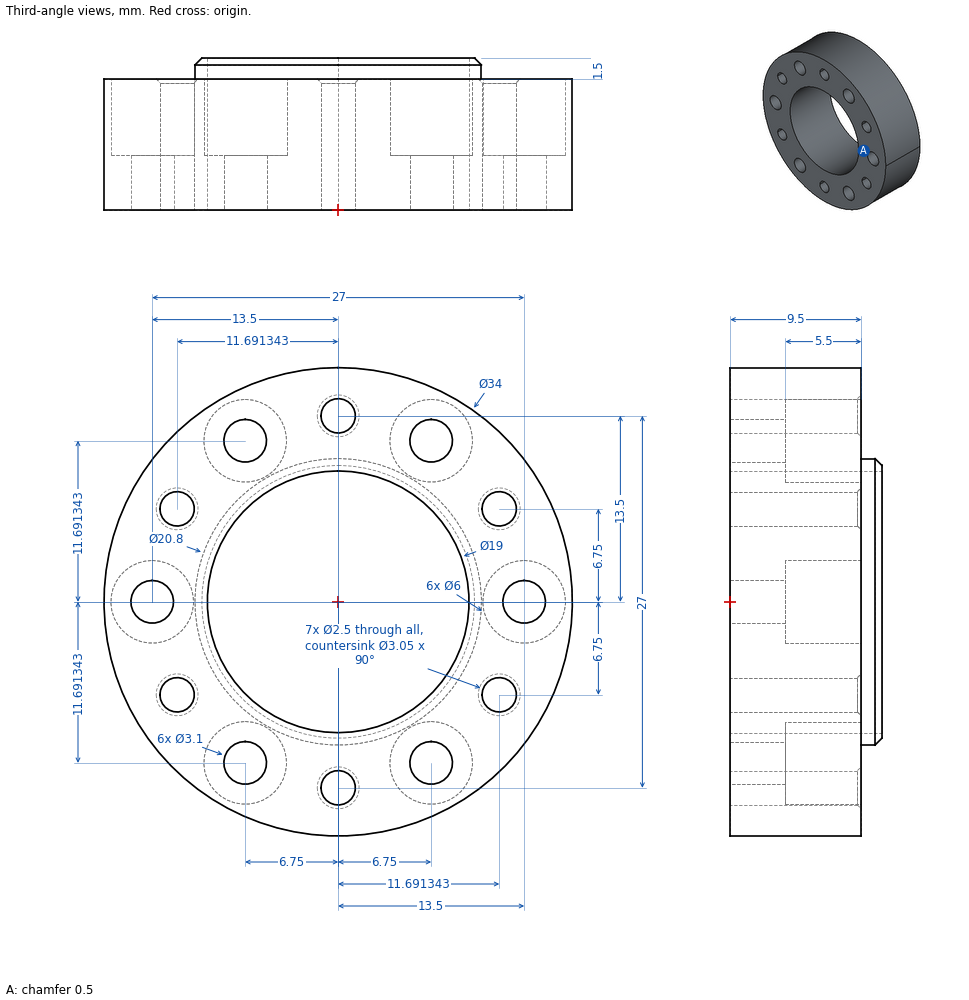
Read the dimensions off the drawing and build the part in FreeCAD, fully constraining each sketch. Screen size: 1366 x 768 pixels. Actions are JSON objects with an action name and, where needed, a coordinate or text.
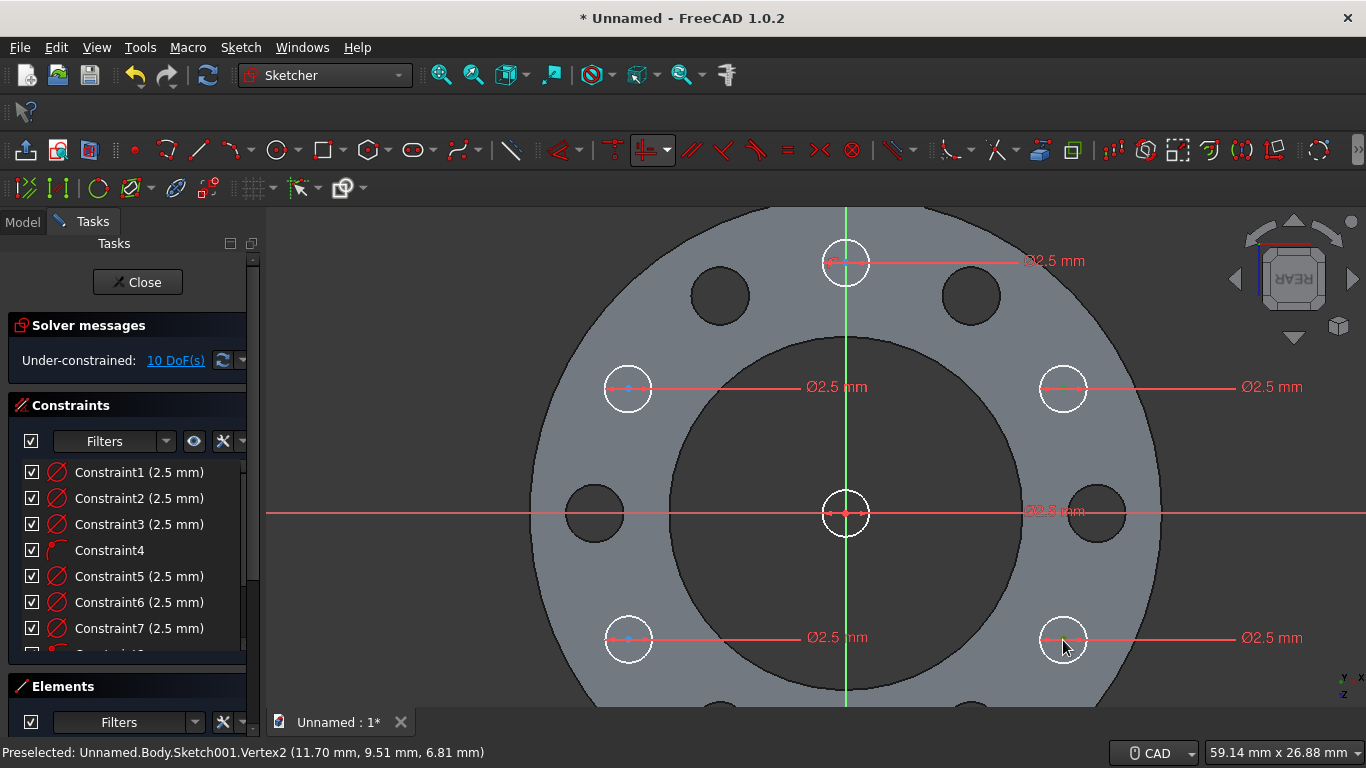
{"action": "left_click", "coordinate": [670, 150]}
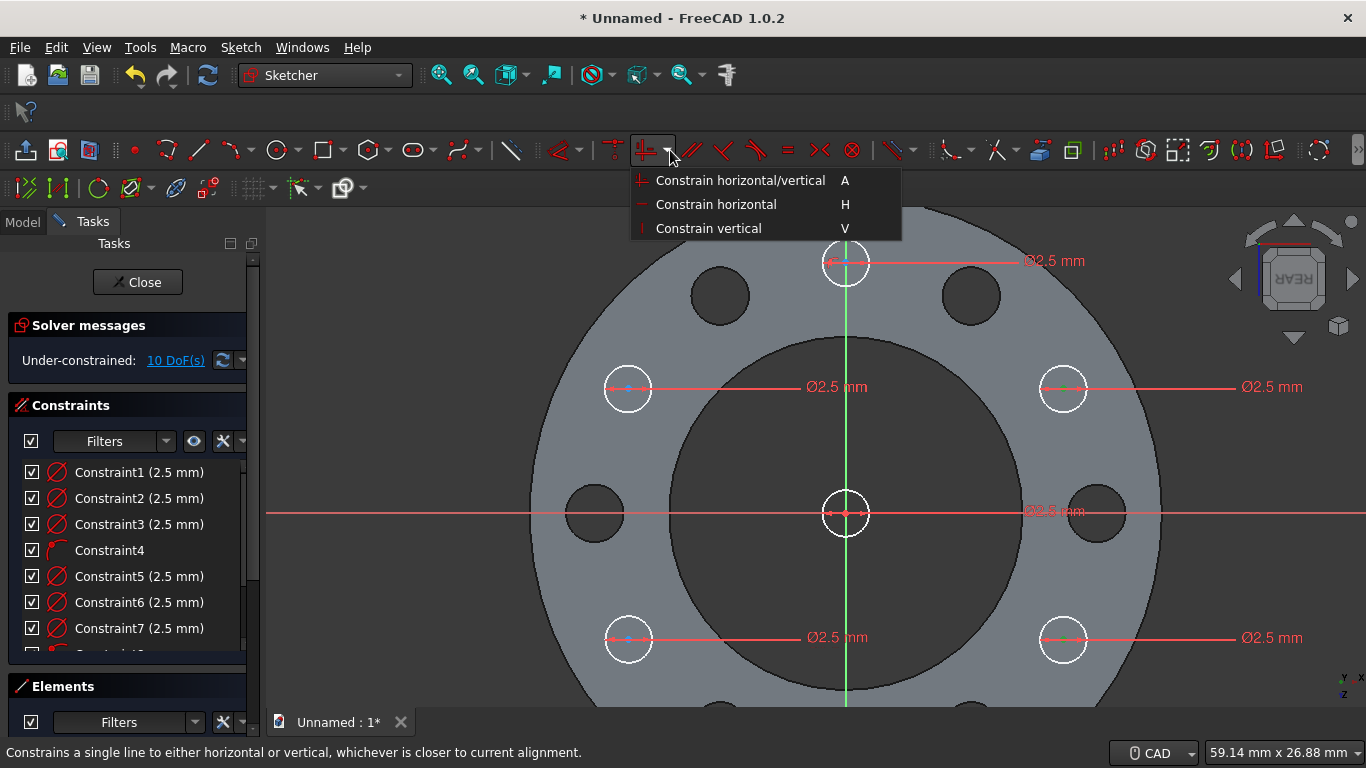
{"action": "left_click", "coordinate": [766, 228]}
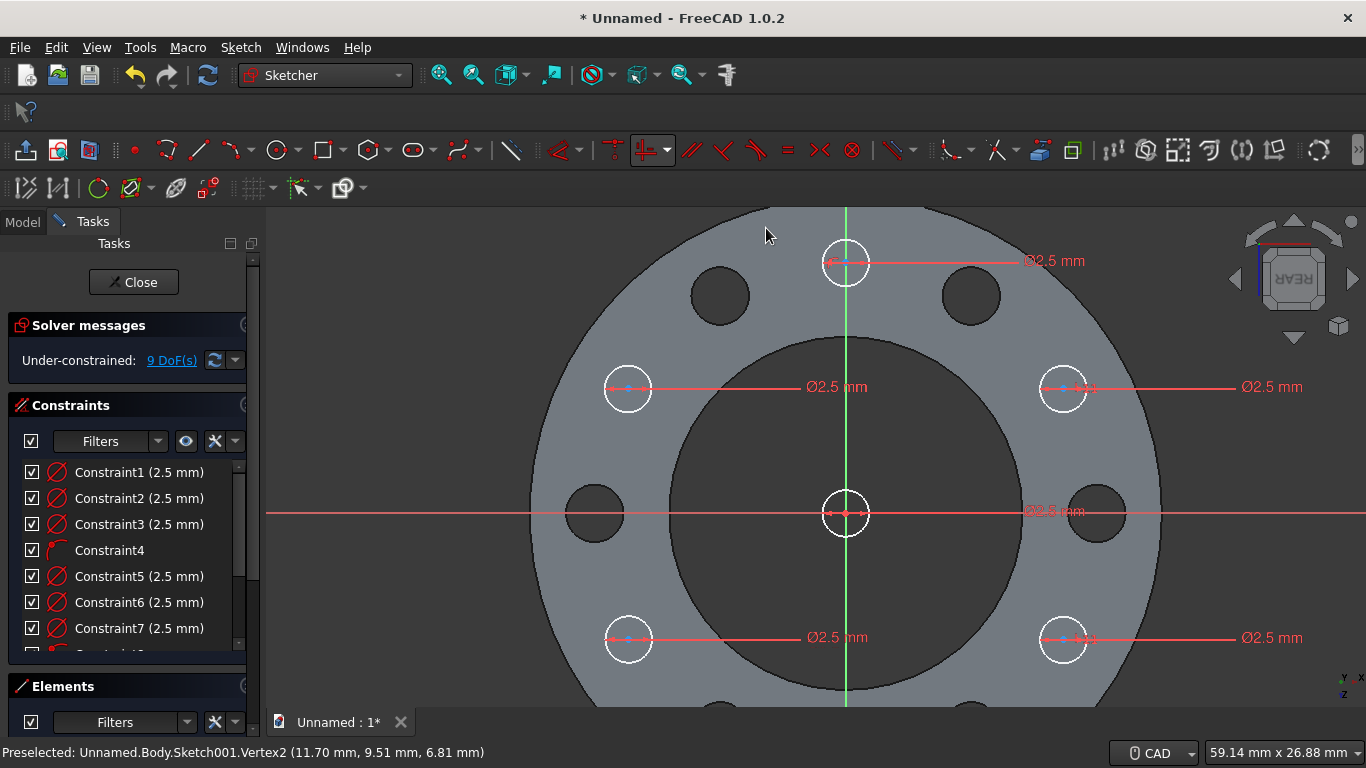
{"action": "left_click", "coordinate": [1063, 640]}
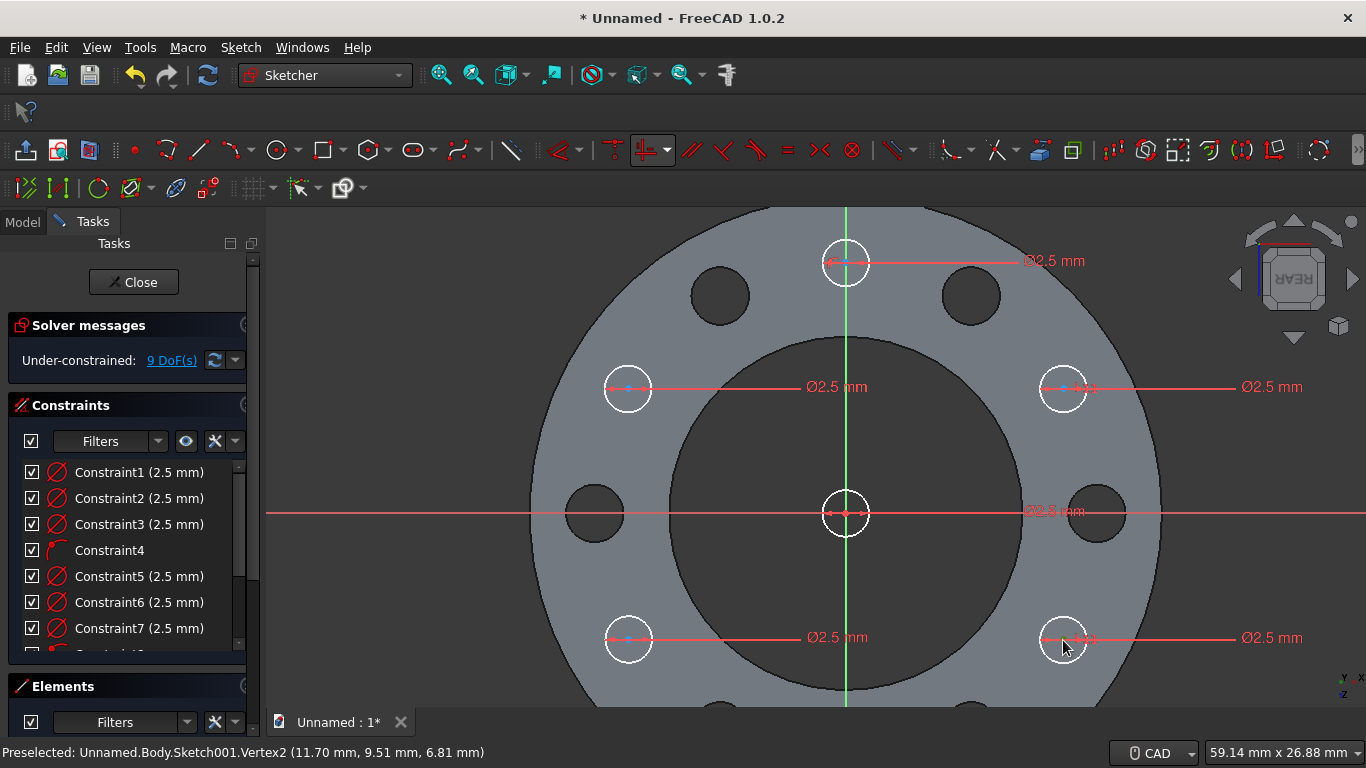
{"action": "left_click", "coordinate": [629, 640]}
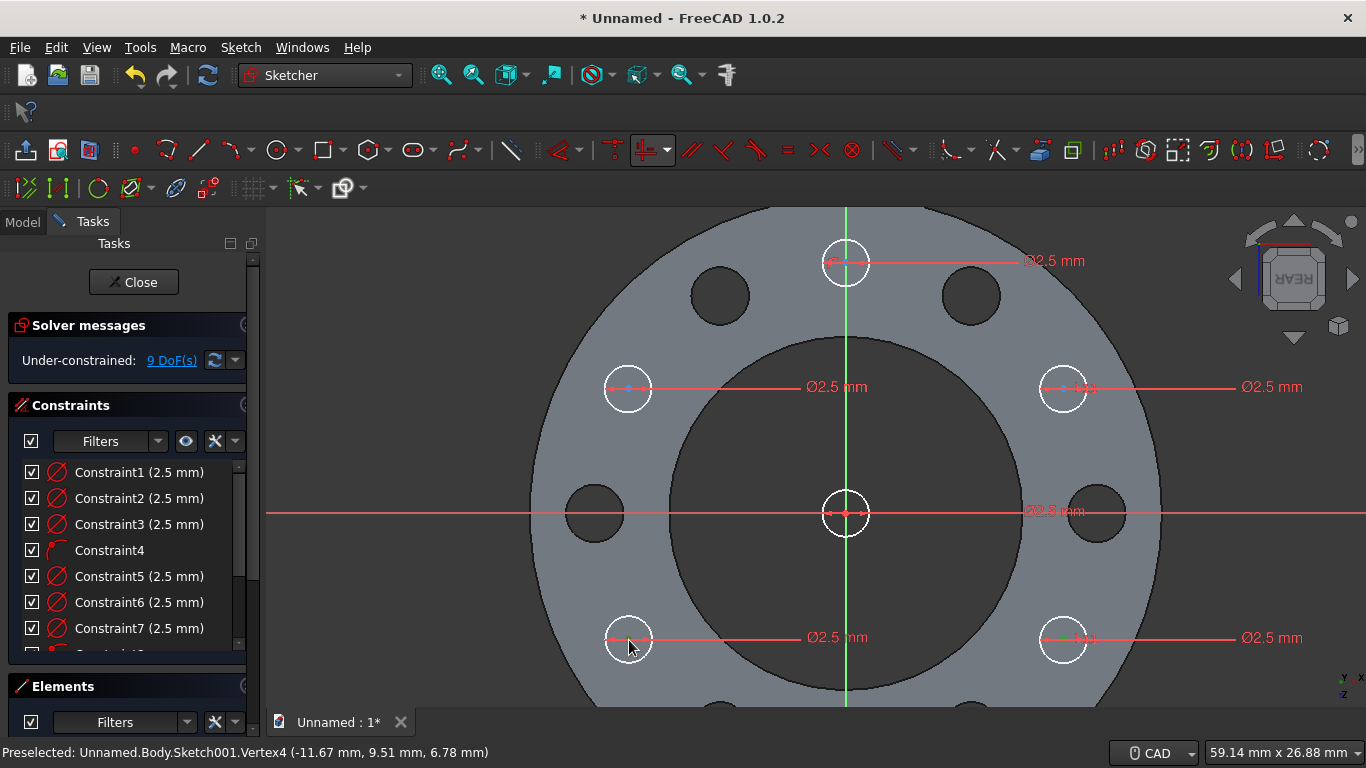
{"action": "left_click", "coordinate": [670, 150]}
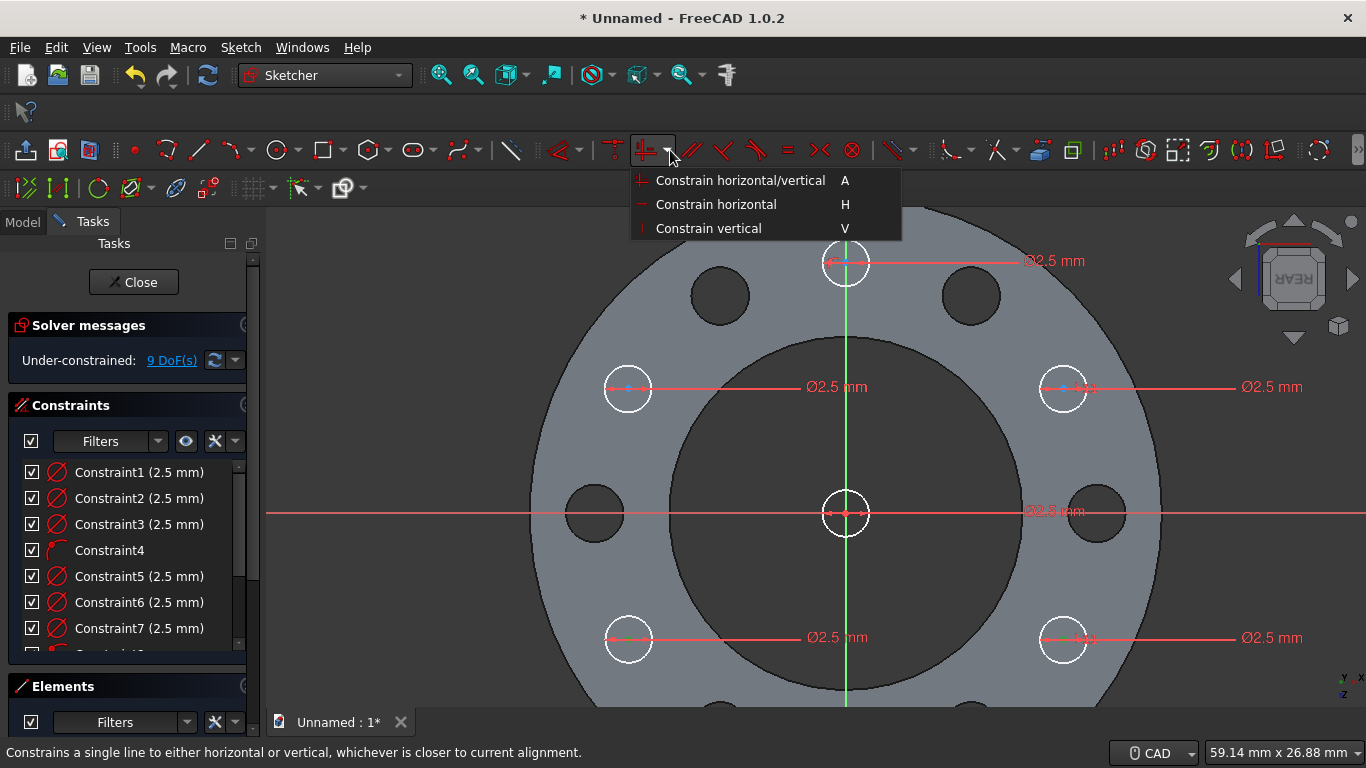
{"action": "left_click", "coordinate": [766, 204]}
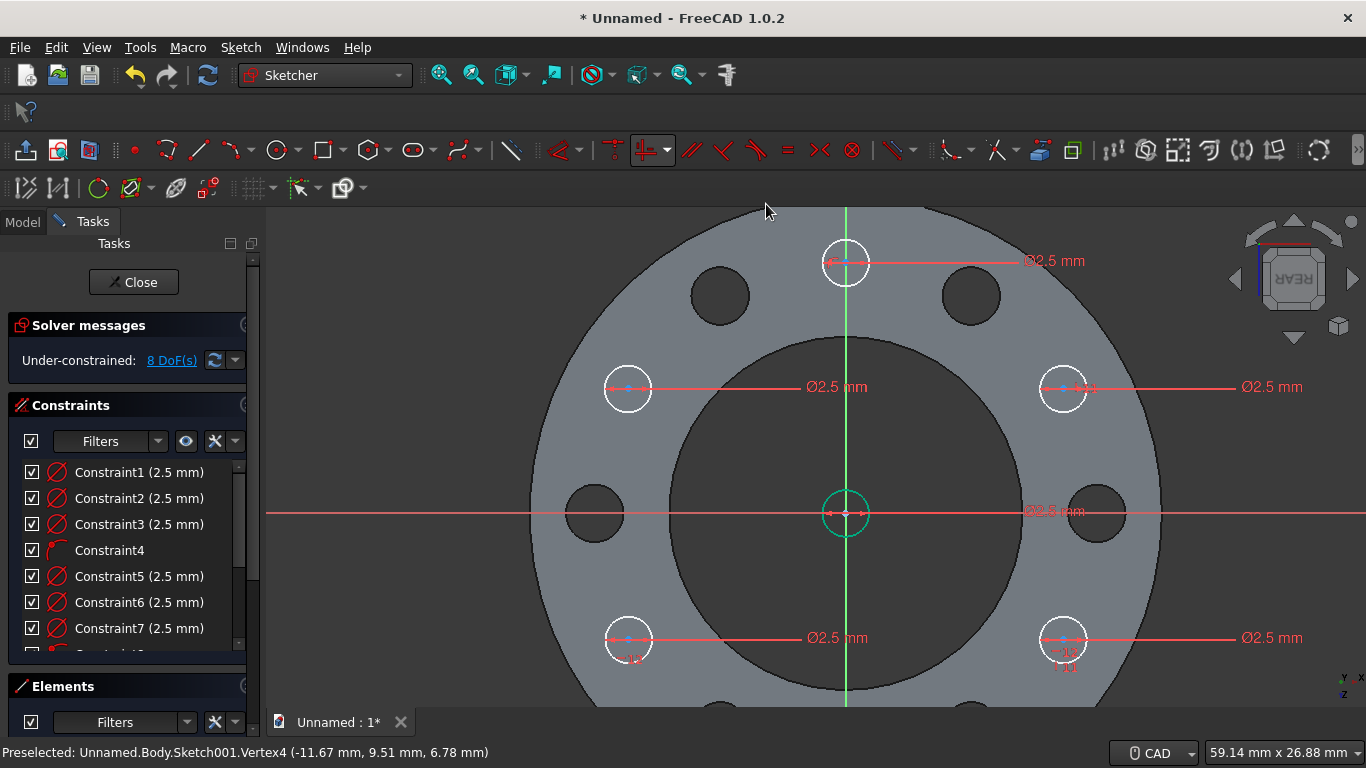
{"action": "left_click", "coordinate": [629, 640]}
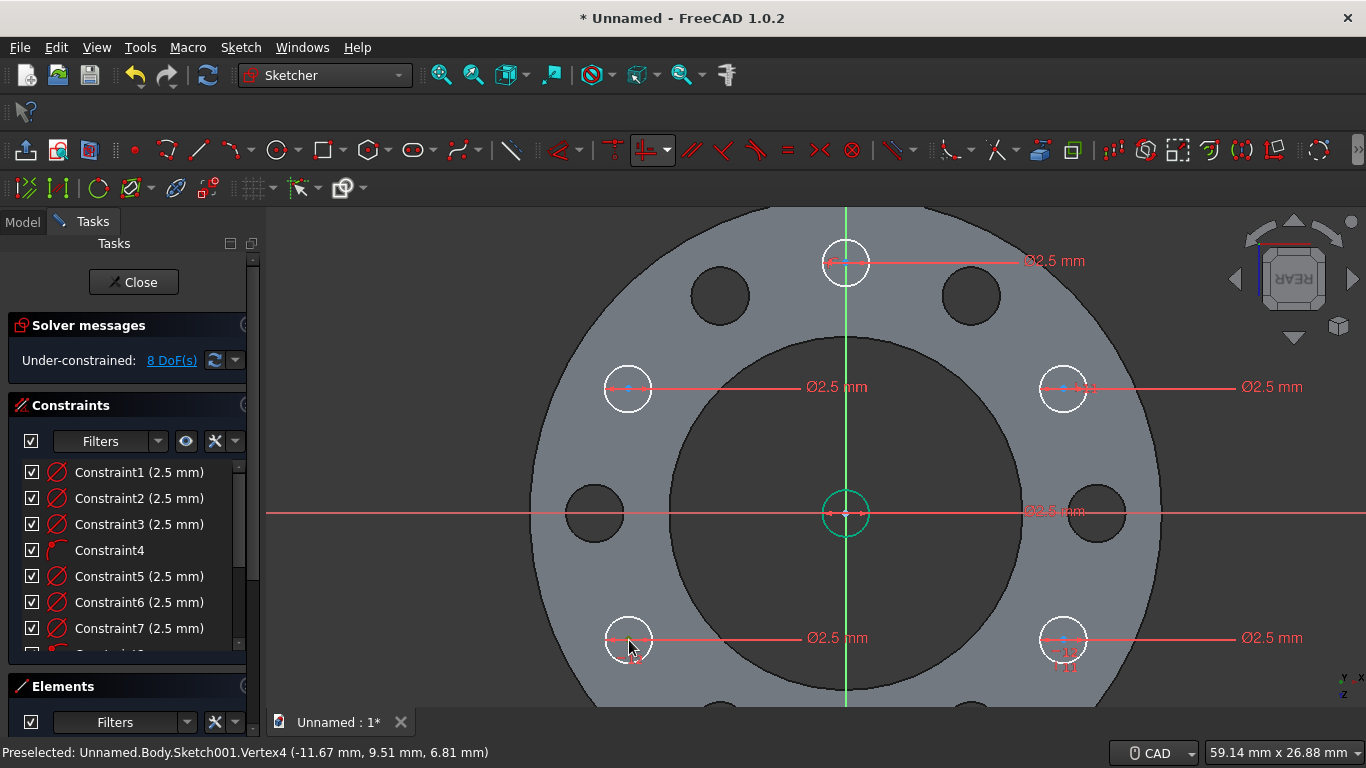
{"action": "left_click", "coordinate": [628, 389]}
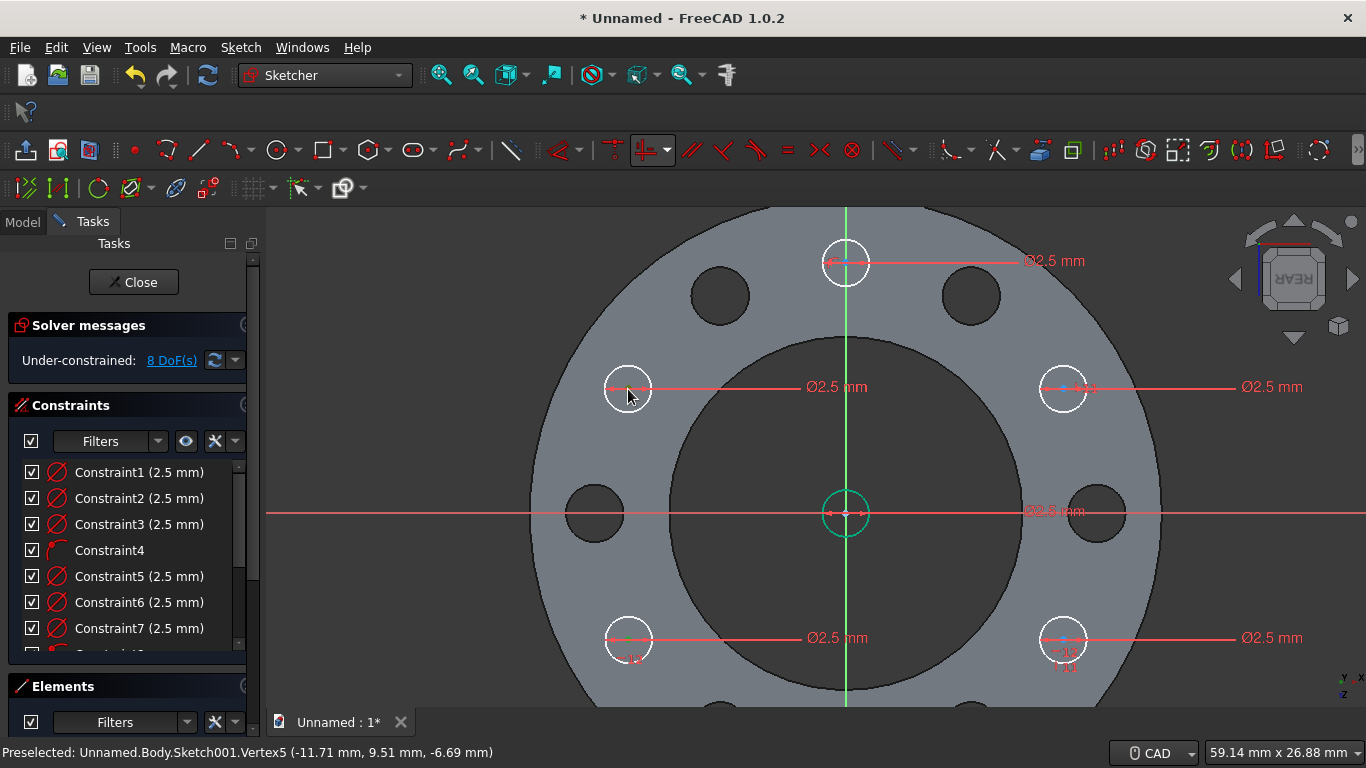
{"action": "key", "text": "v"}